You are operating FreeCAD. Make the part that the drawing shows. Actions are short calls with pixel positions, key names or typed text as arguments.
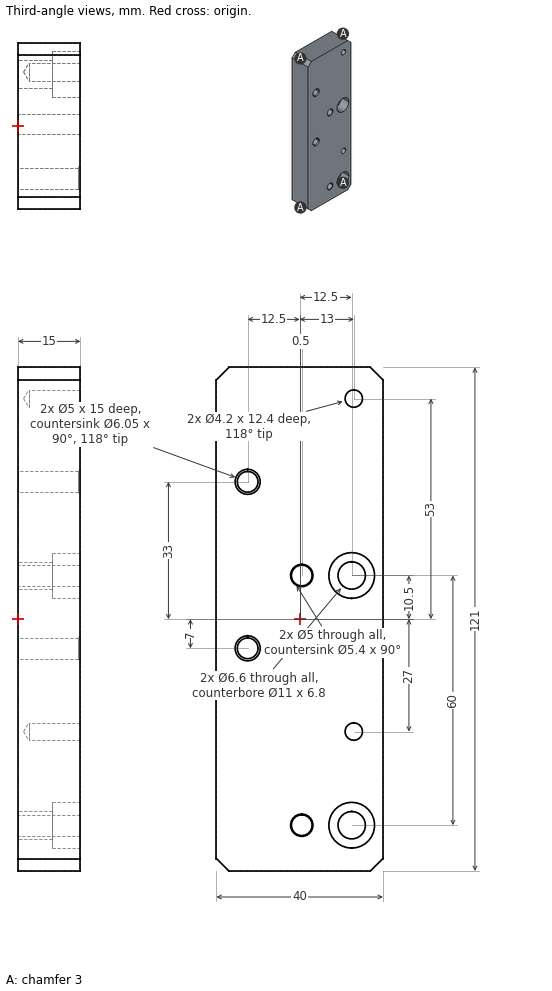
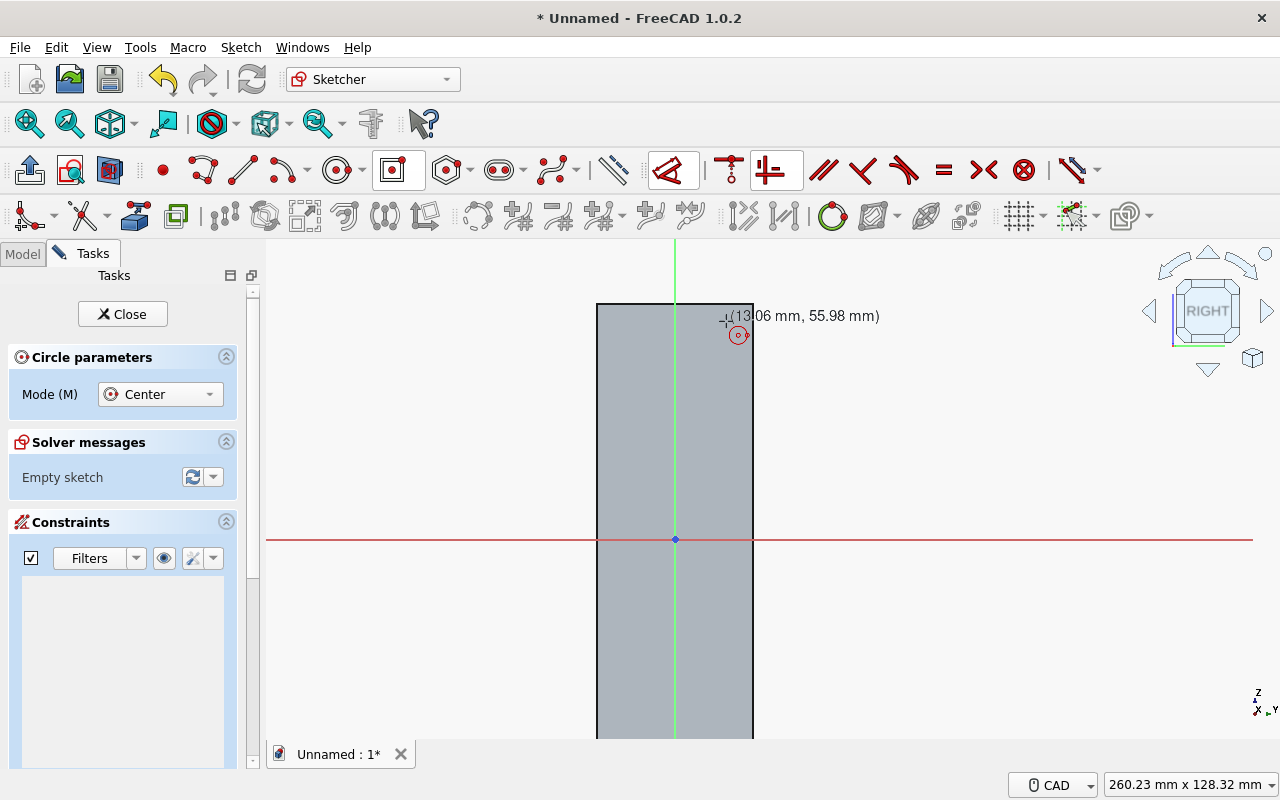
click(726, 333)
move(732, 327)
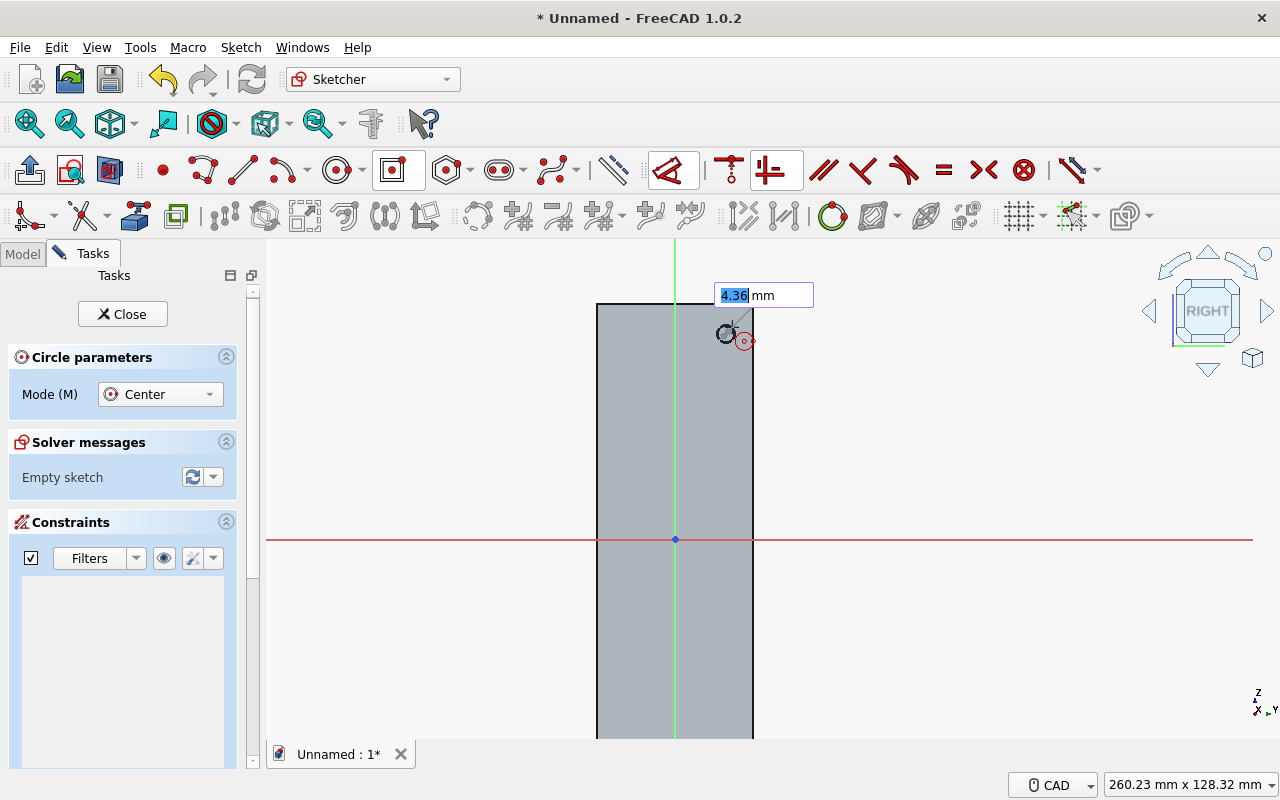
text(4.2)
key(Return)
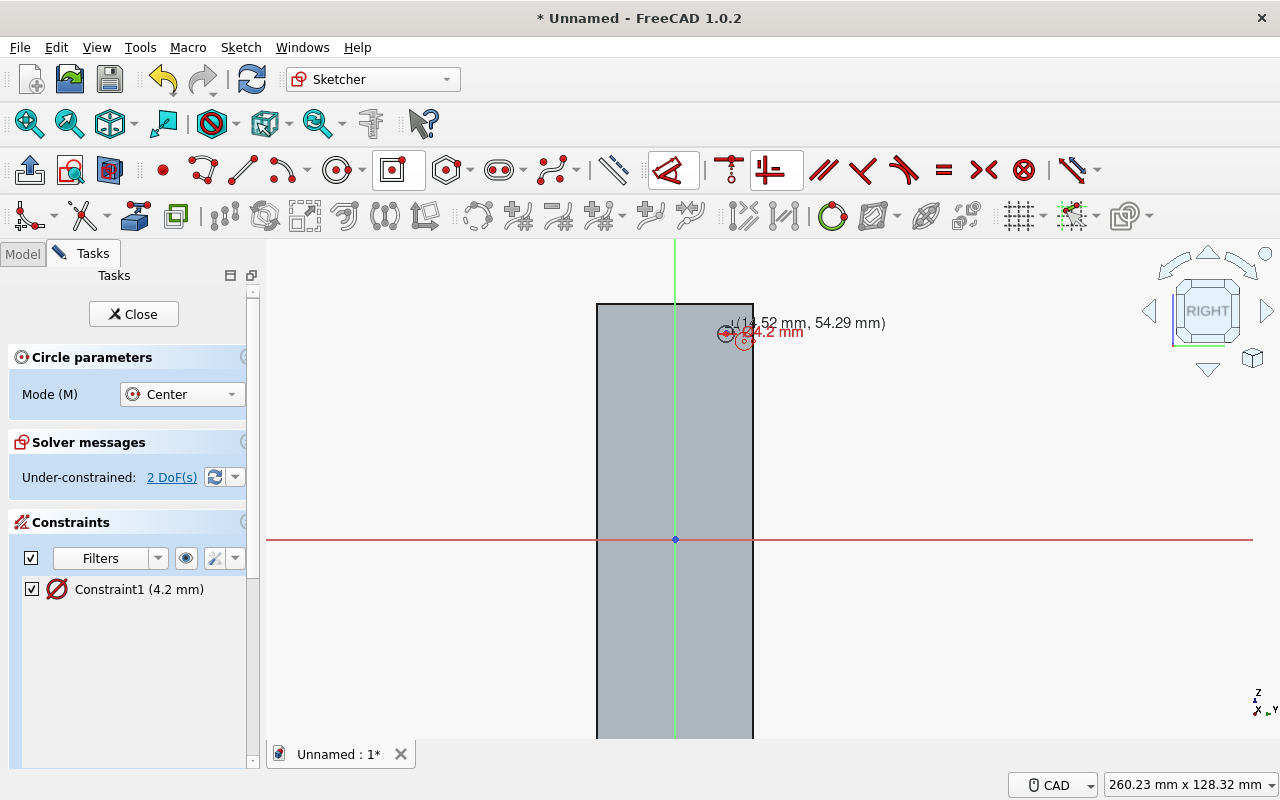
scroll(726, 645, up, 6)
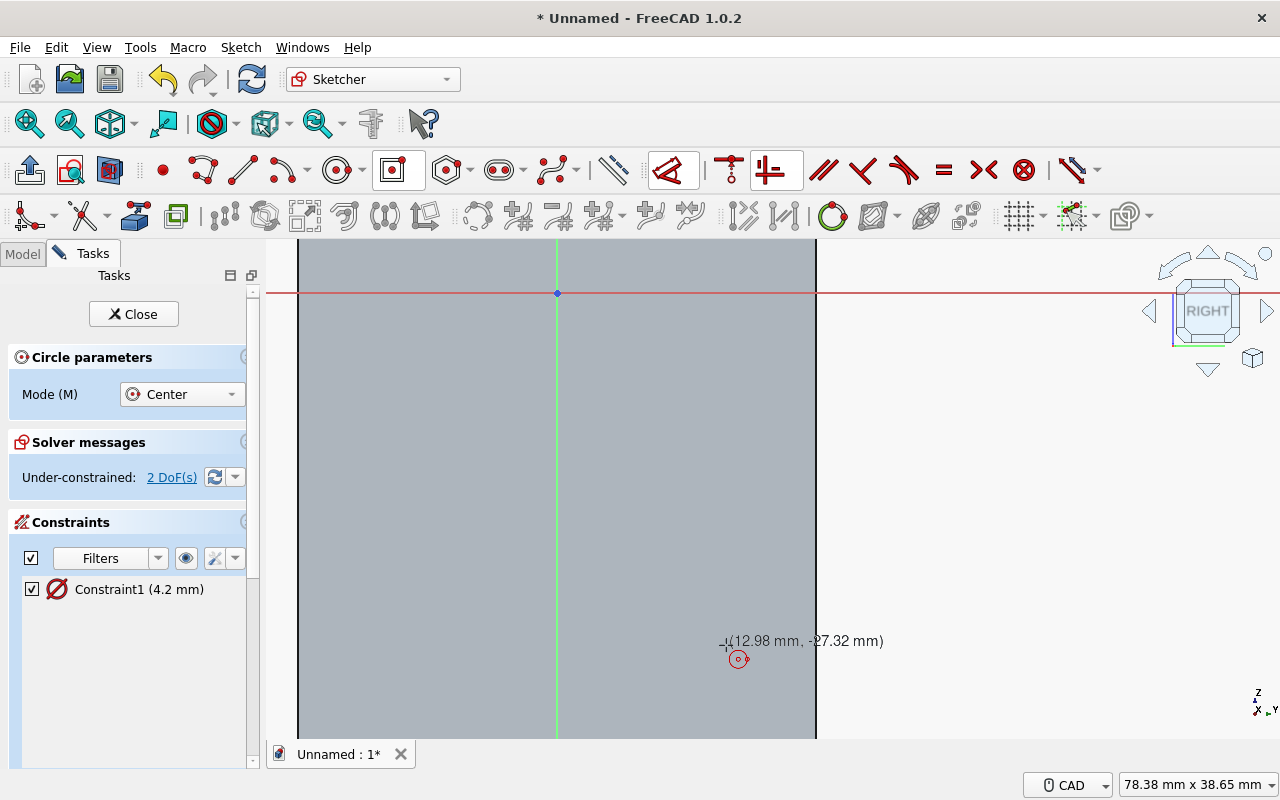
scroll(726, 646, down, 6)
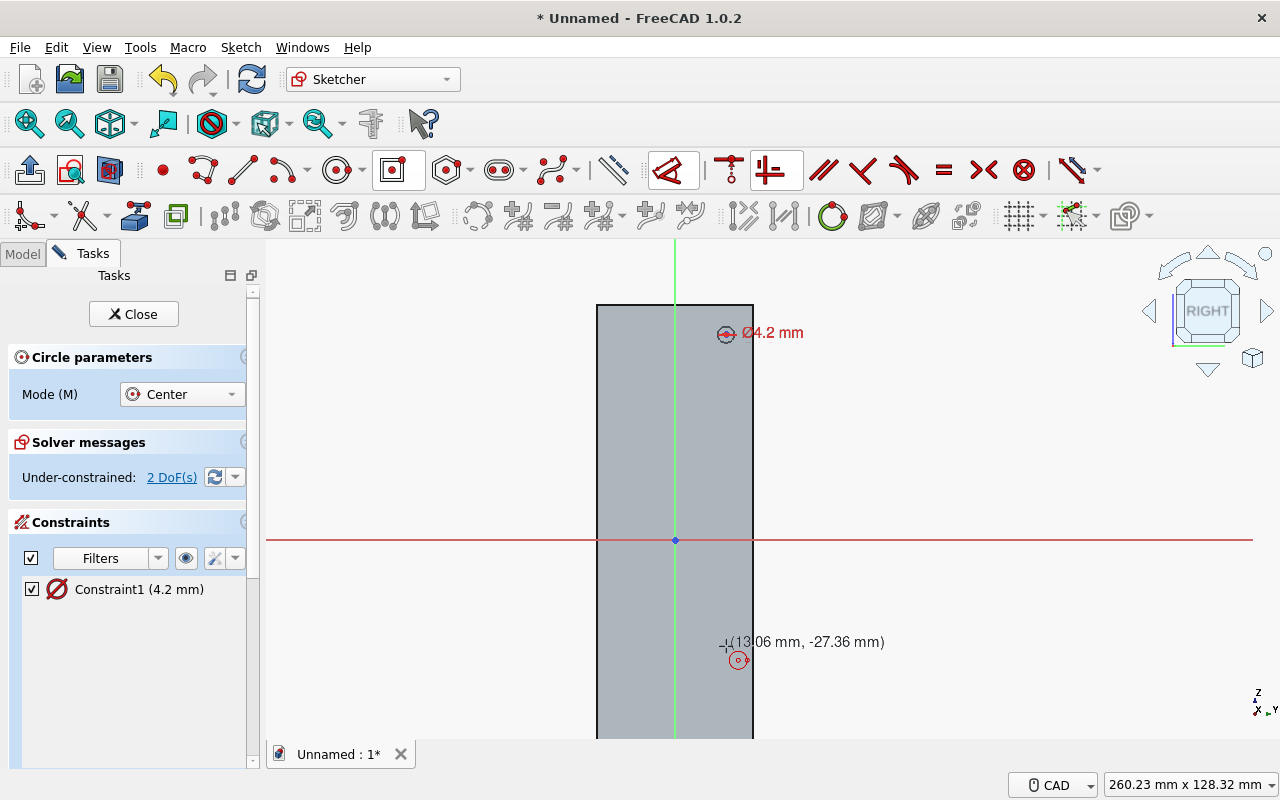
click(726, 645)
move(732, 640)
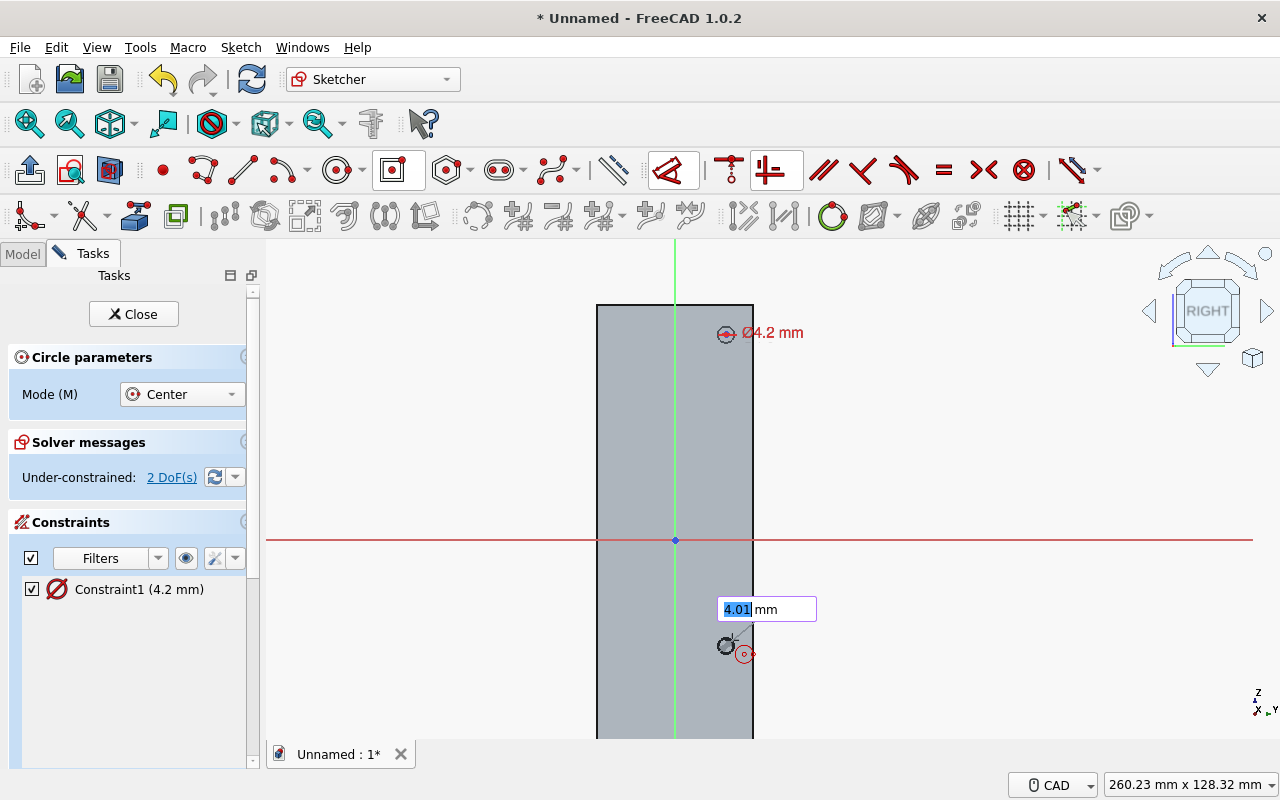
text(4.2)
key(Return)
key(Escape)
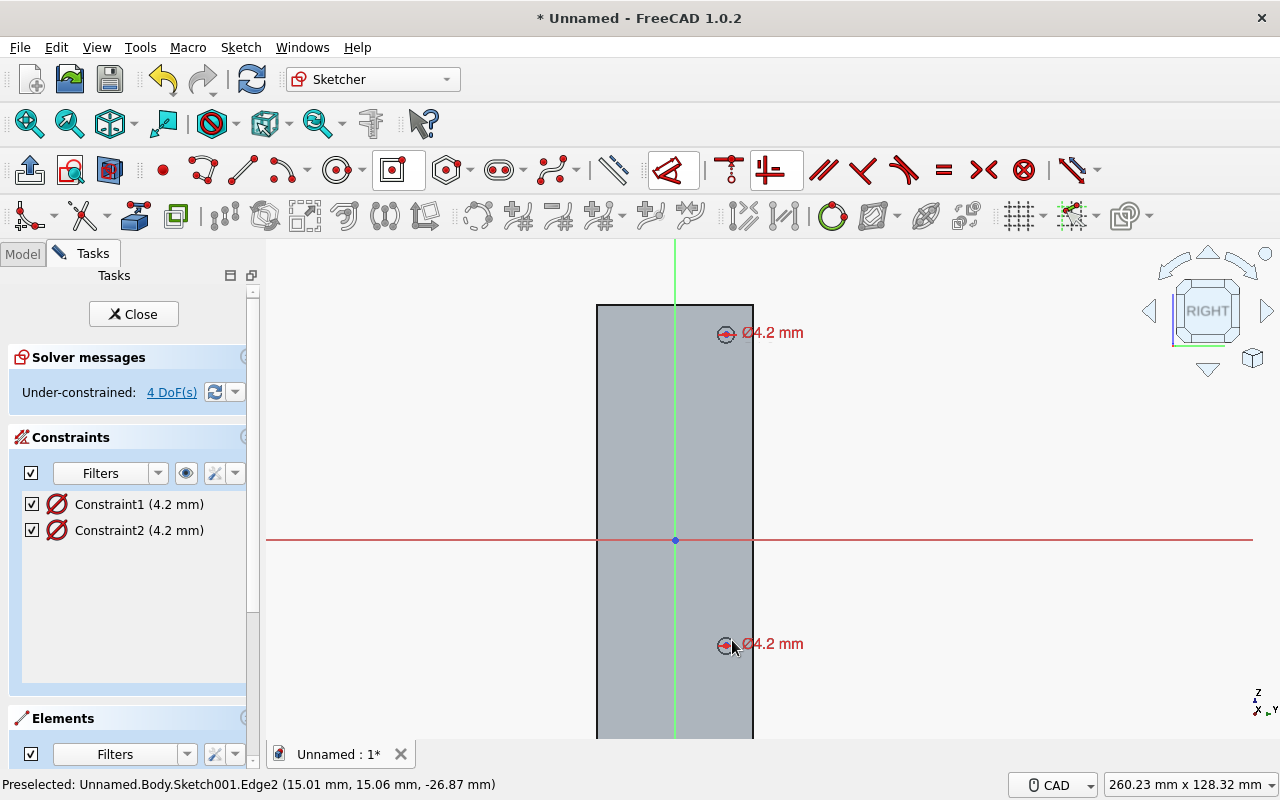
click(726, 335)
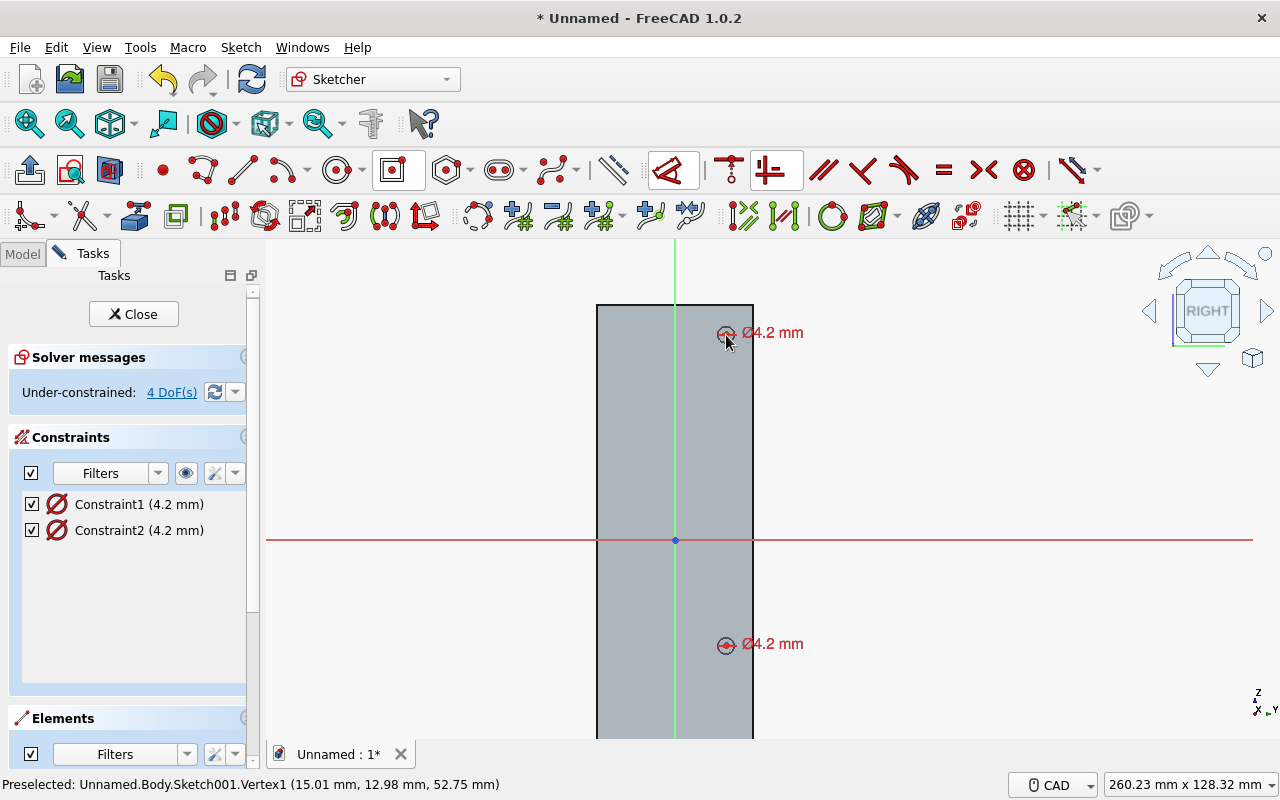
click(726, 646)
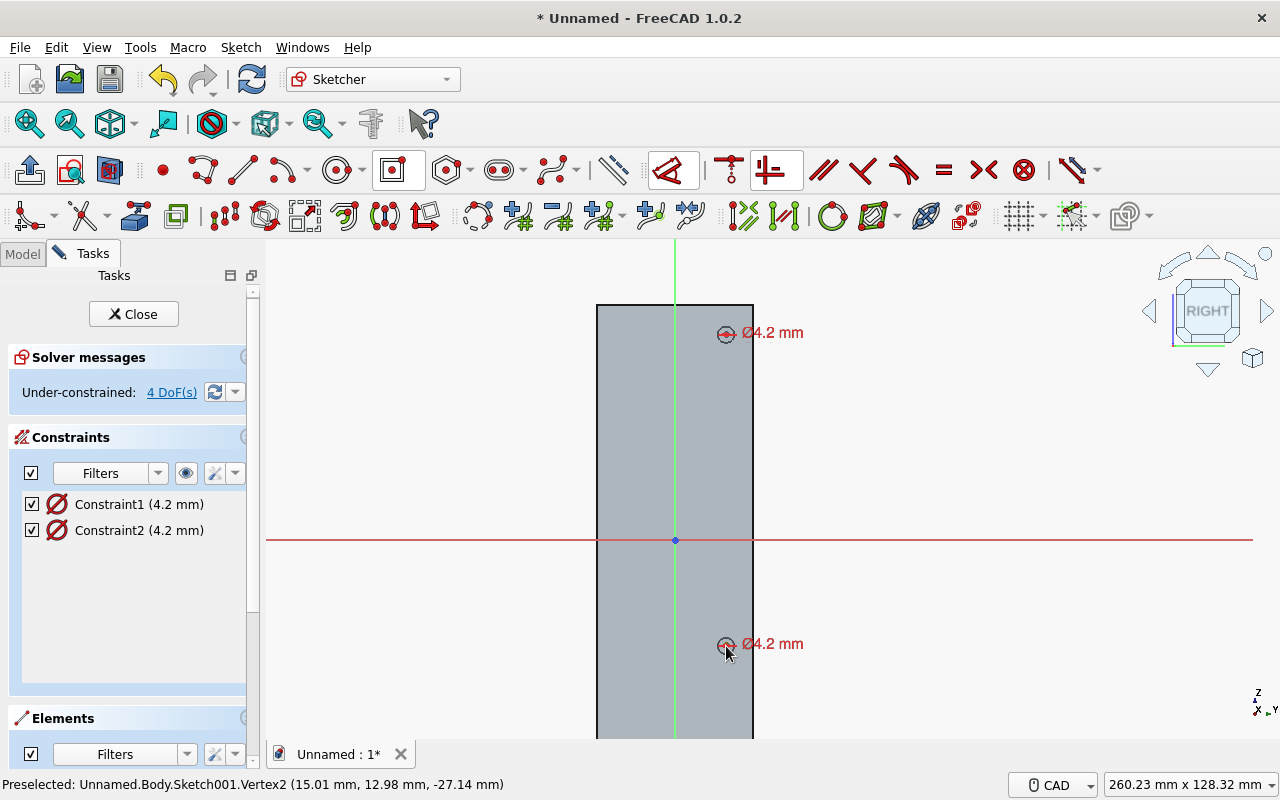
key(v)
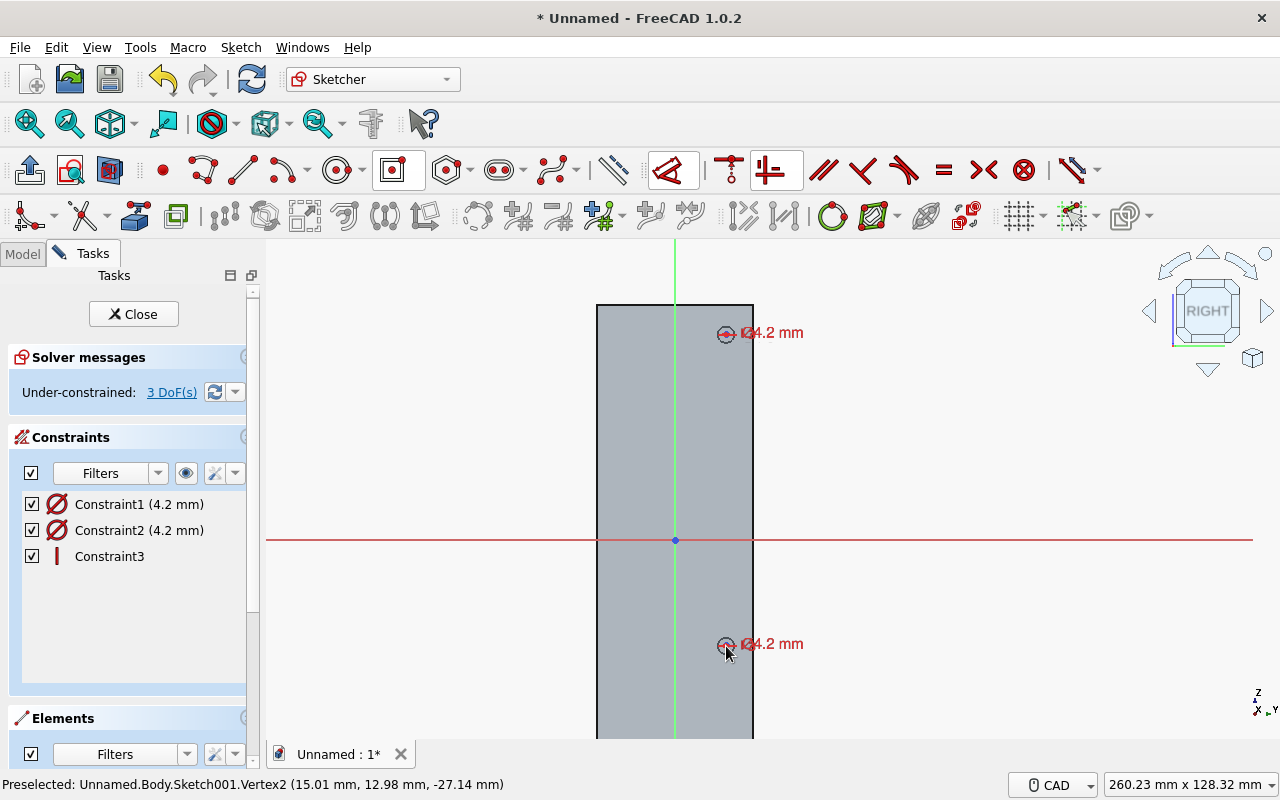
click(726, 335)